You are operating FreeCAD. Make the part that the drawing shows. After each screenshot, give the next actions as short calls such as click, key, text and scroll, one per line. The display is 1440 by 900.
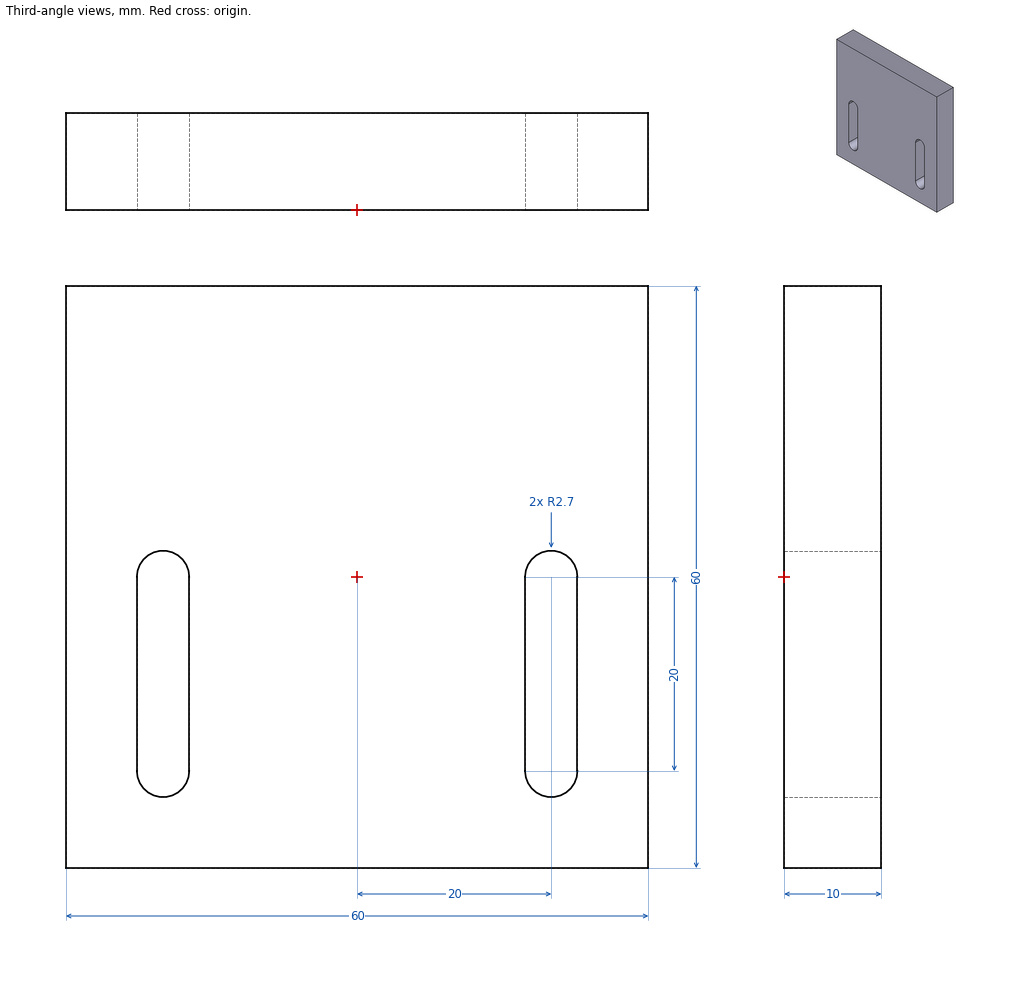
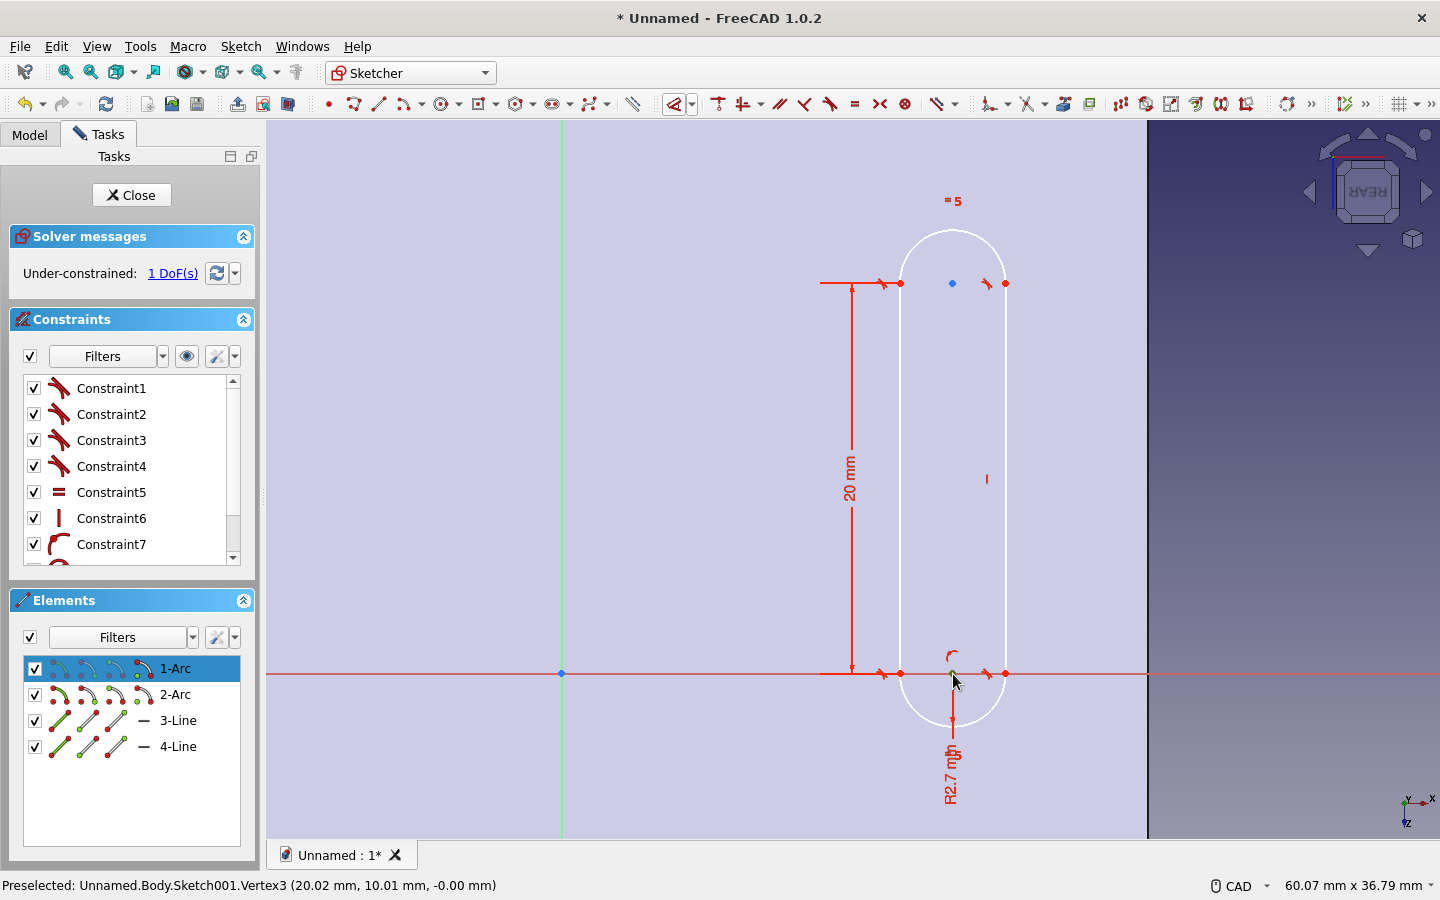
click(692, 104)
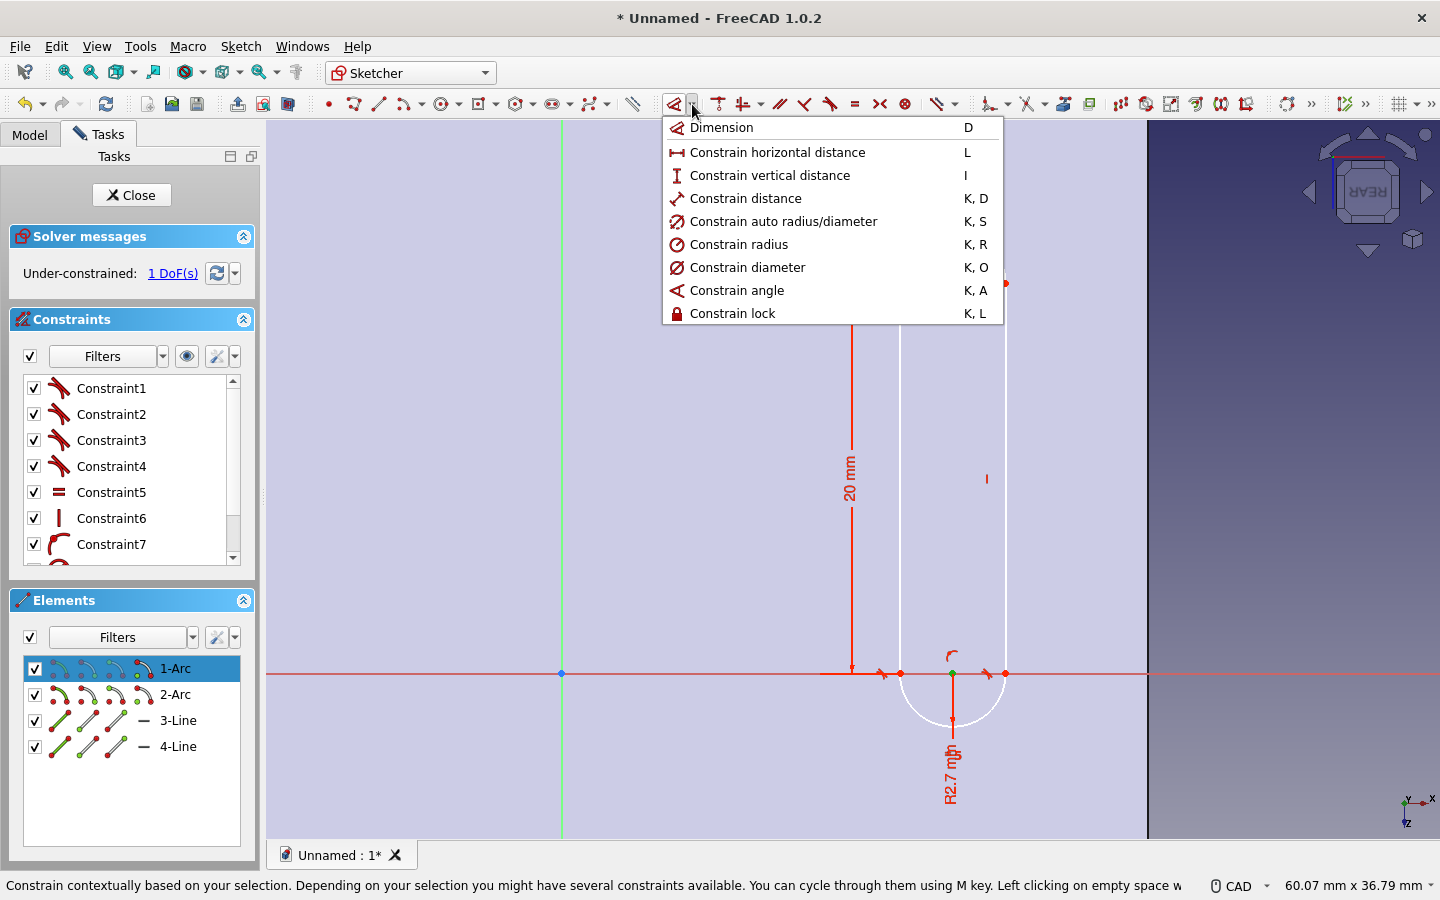
click(833, 152)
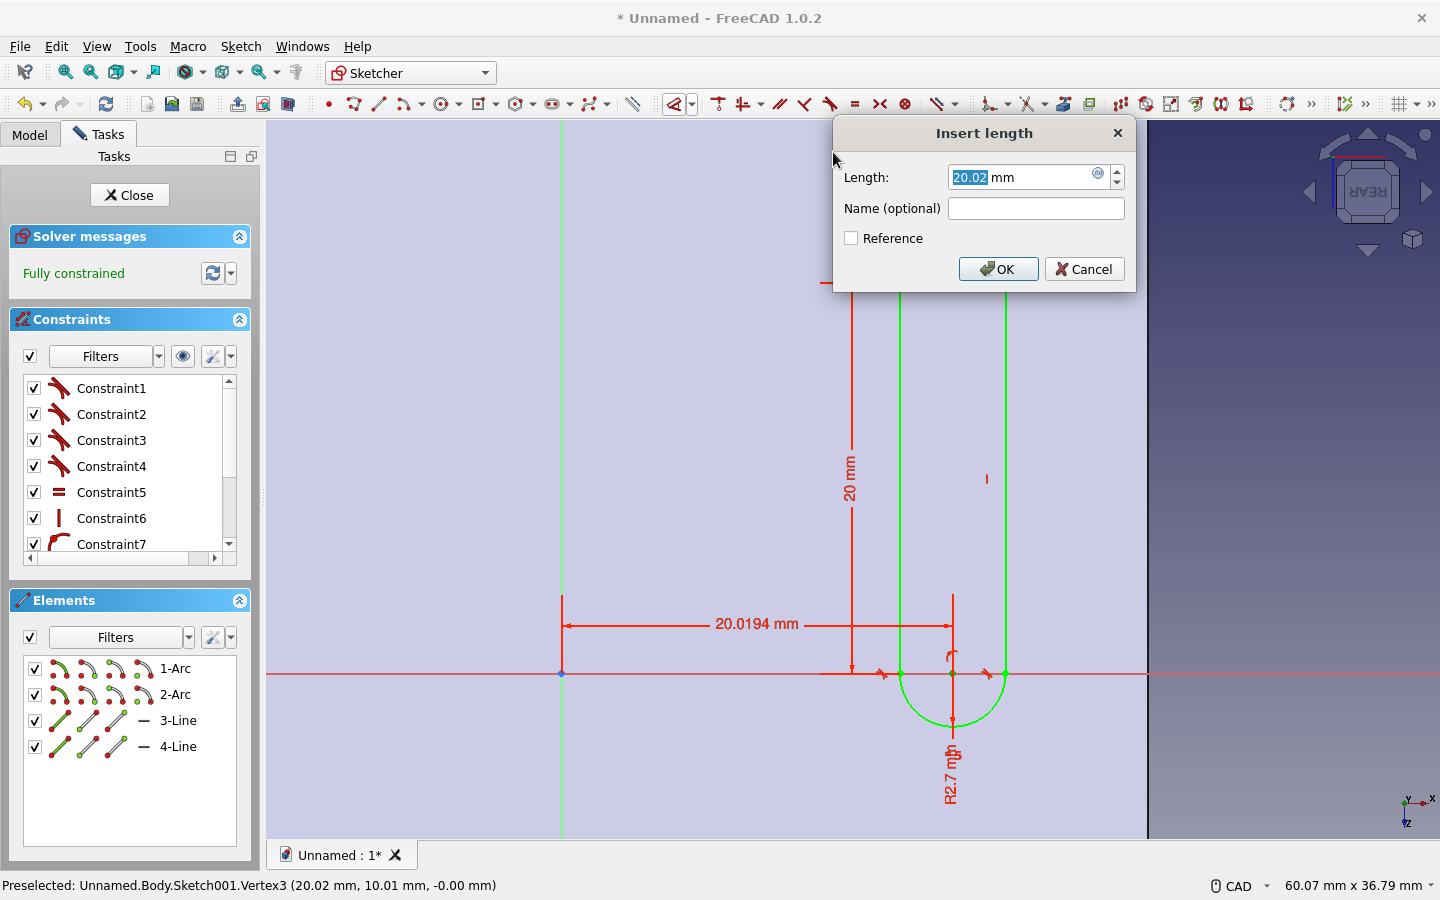
text(20)
key(Return)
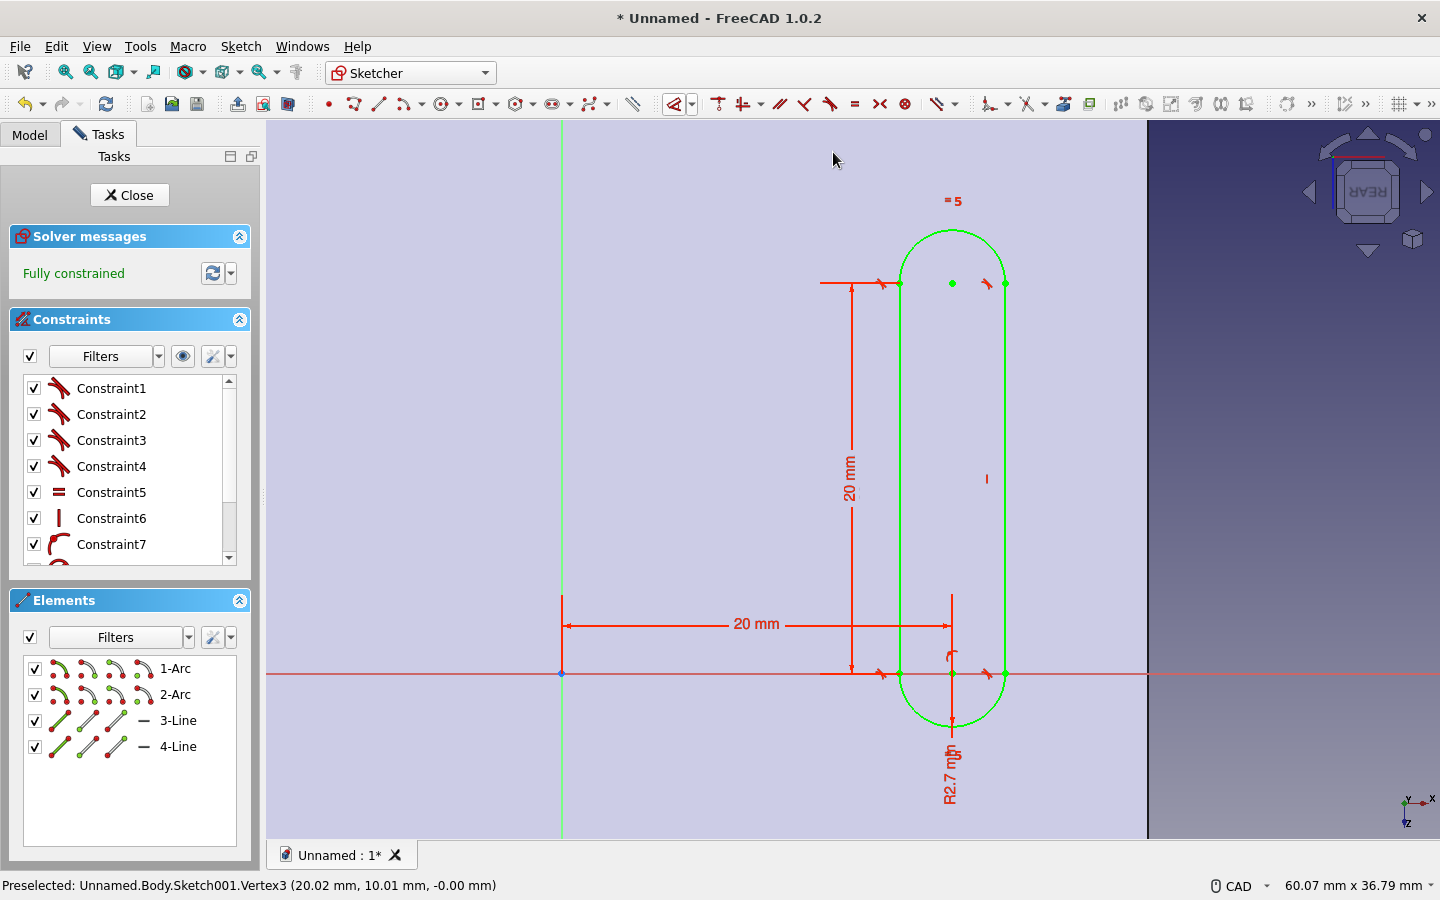
click(130, 195)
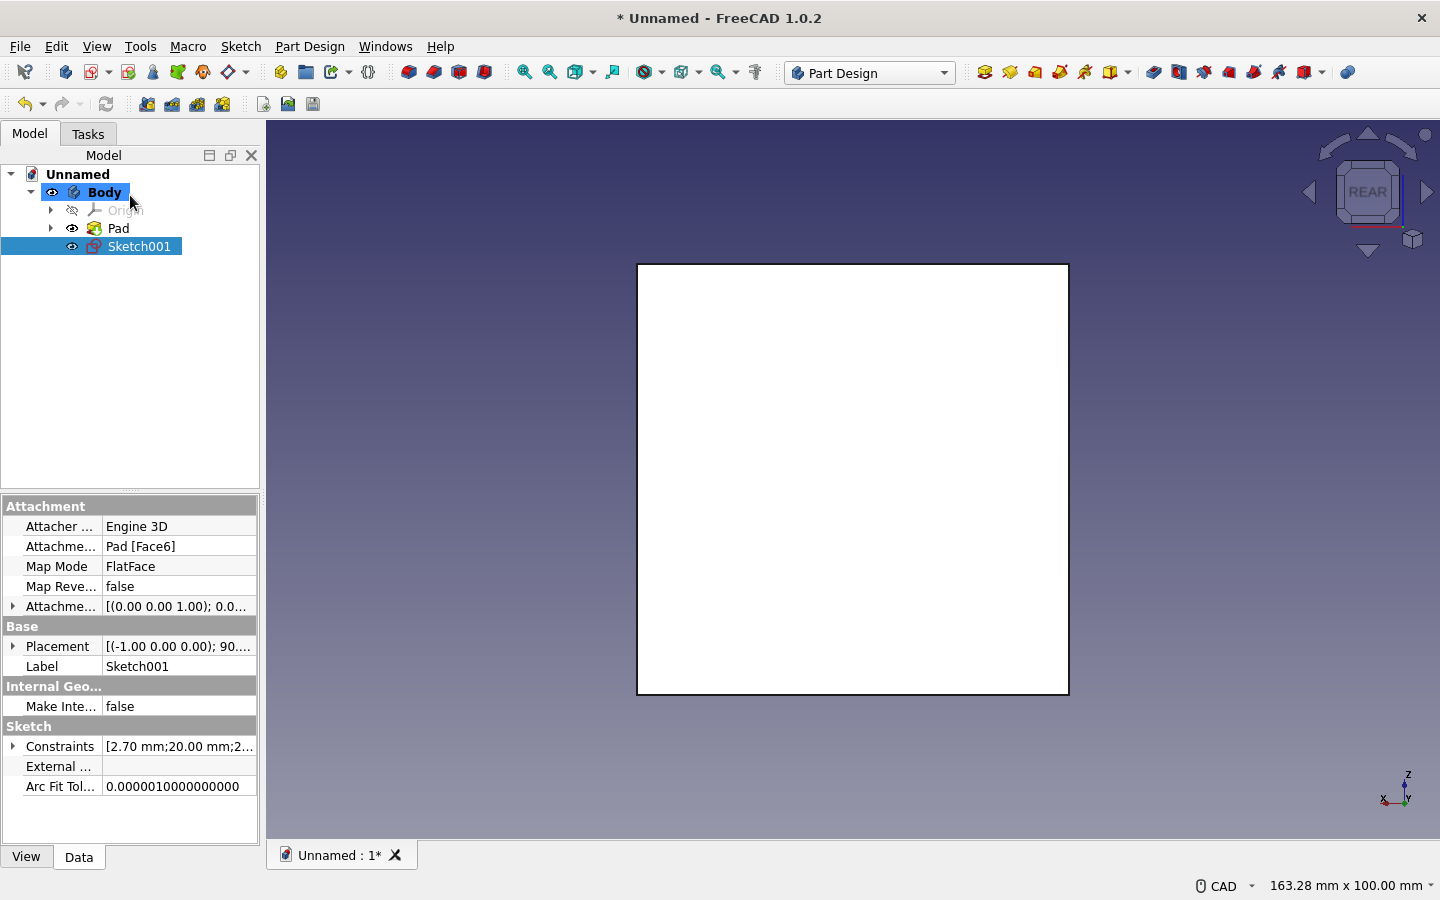
click(1154, 72)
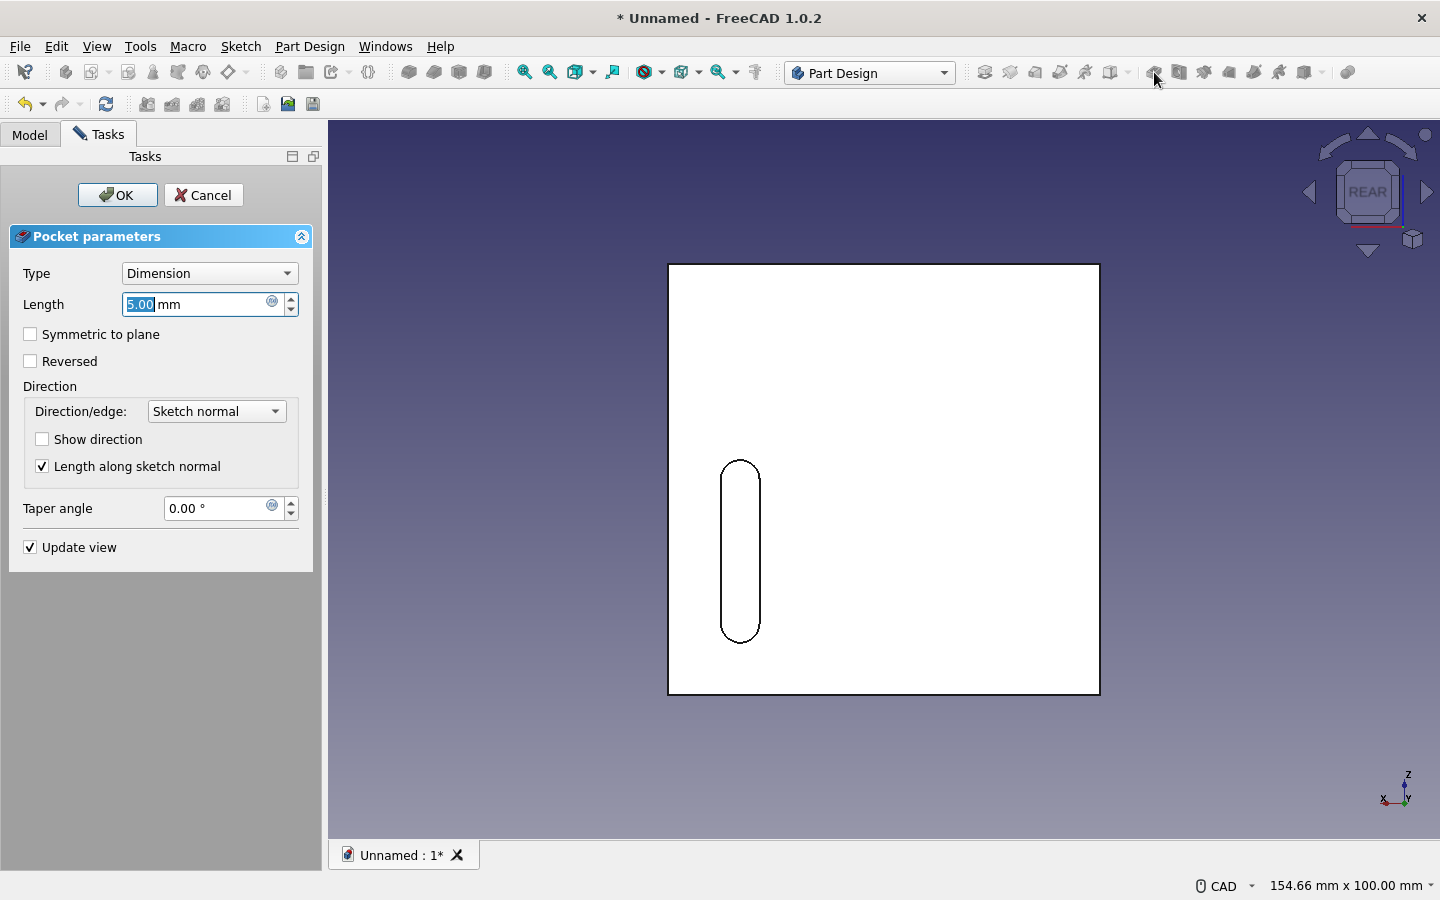
click(210, 274)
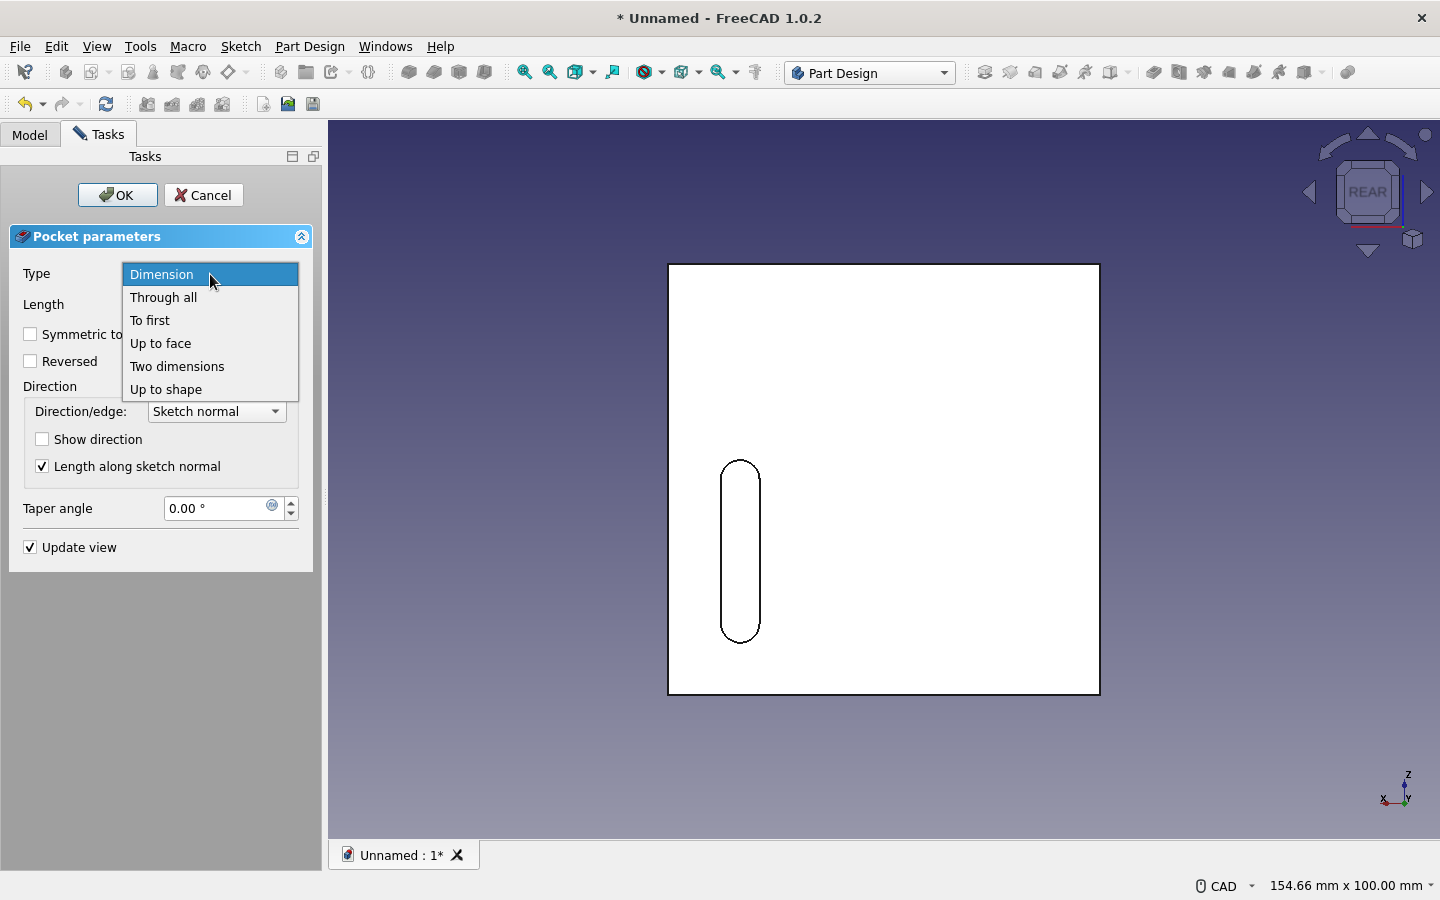
click(208, 298)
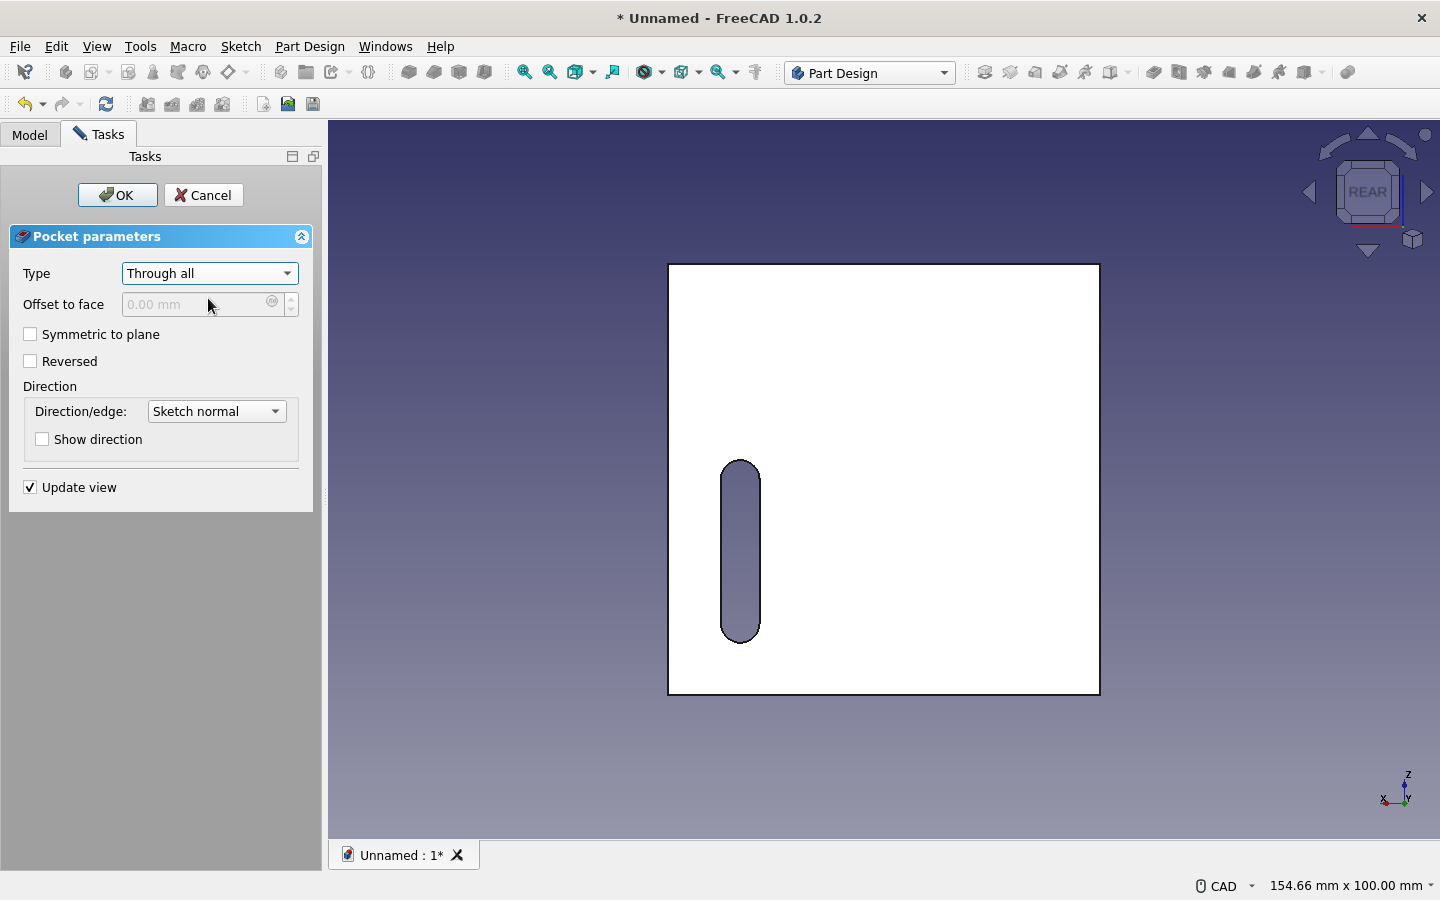
click(118, 195)